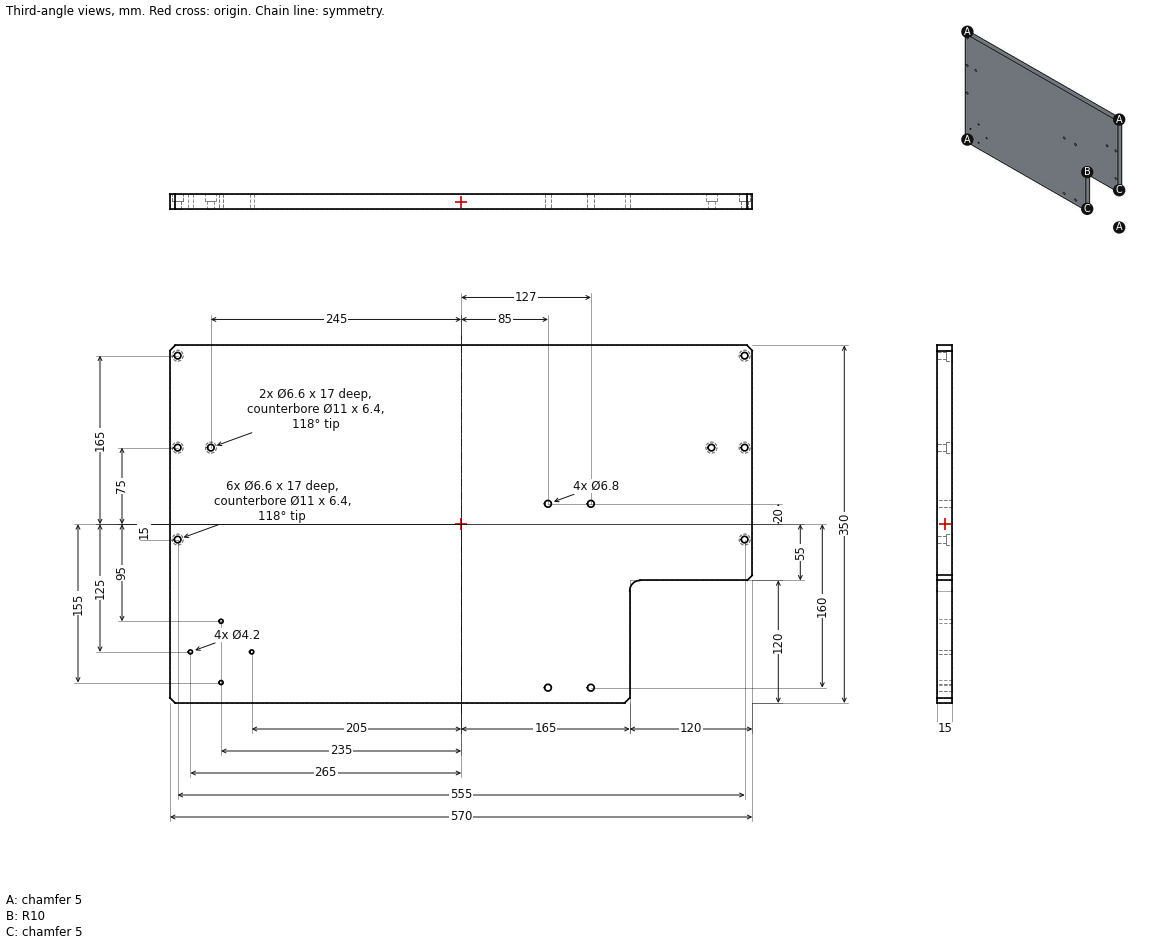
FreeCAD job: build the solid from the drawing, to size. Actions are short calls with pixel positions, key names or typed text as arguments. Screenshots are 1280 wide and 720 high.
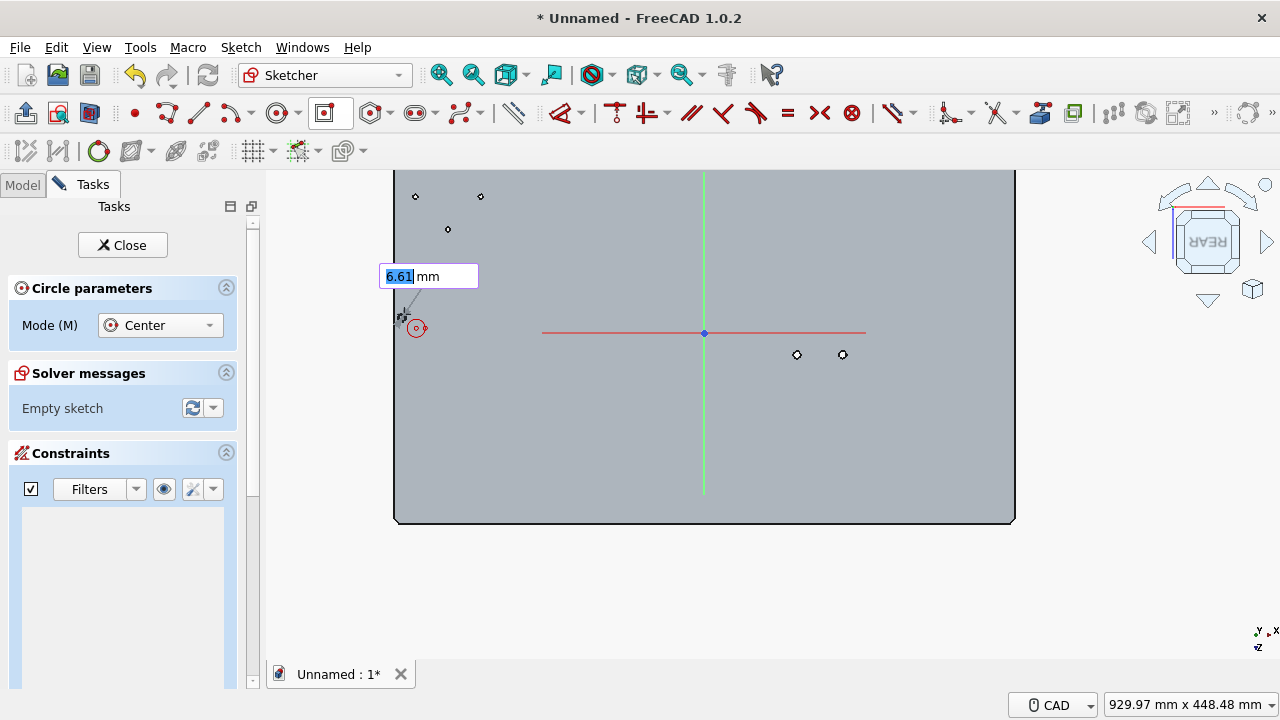
text(6.6)
key(Return)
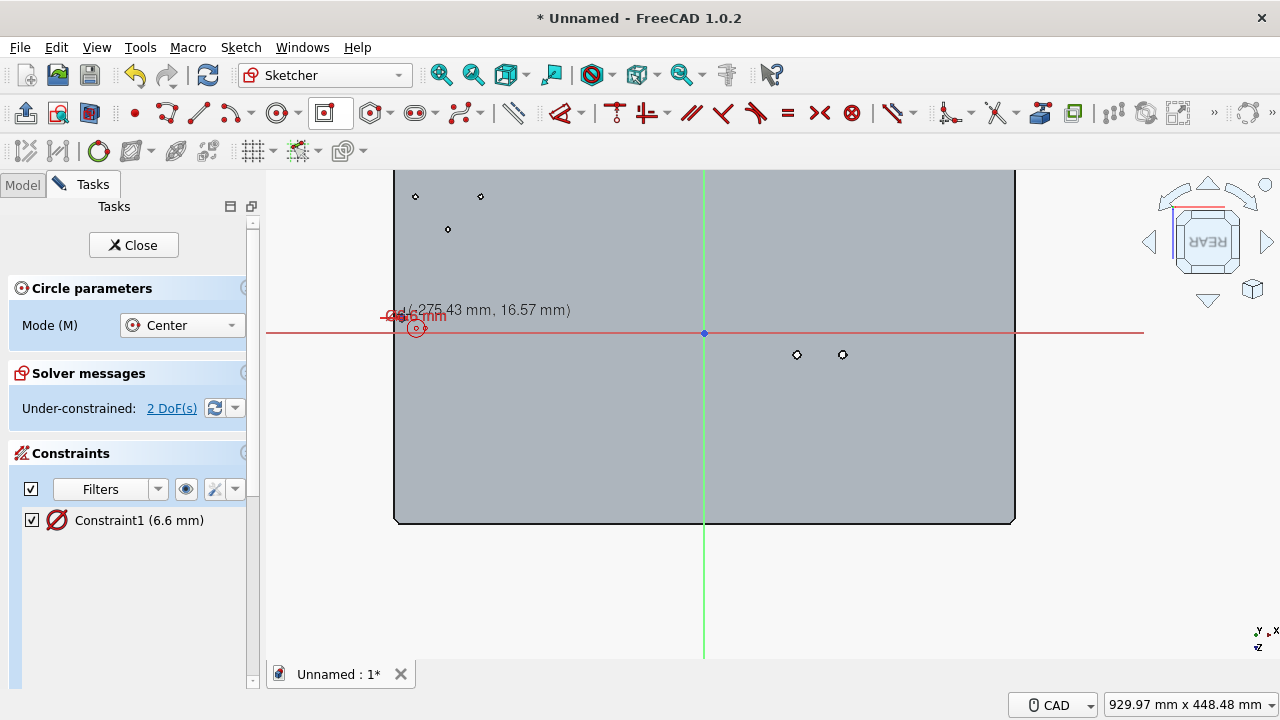
scroll(402, 513, up, 10)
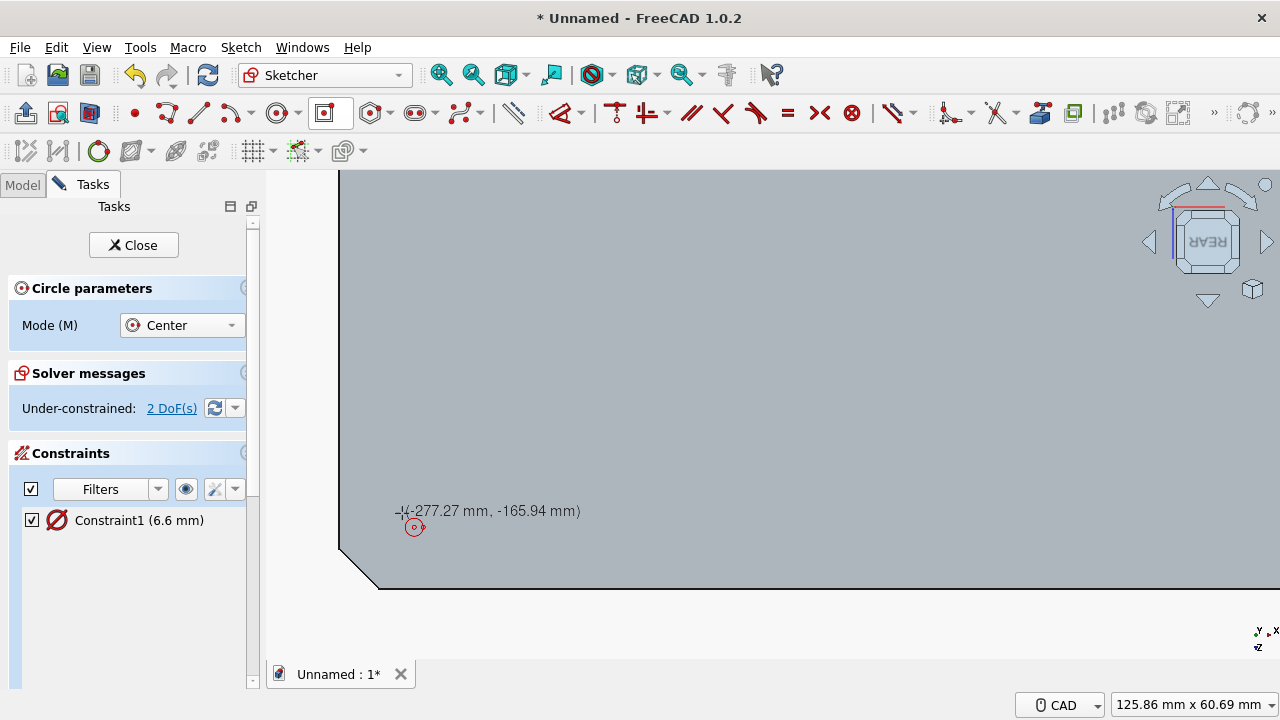
scroll(402, 513, down, 10)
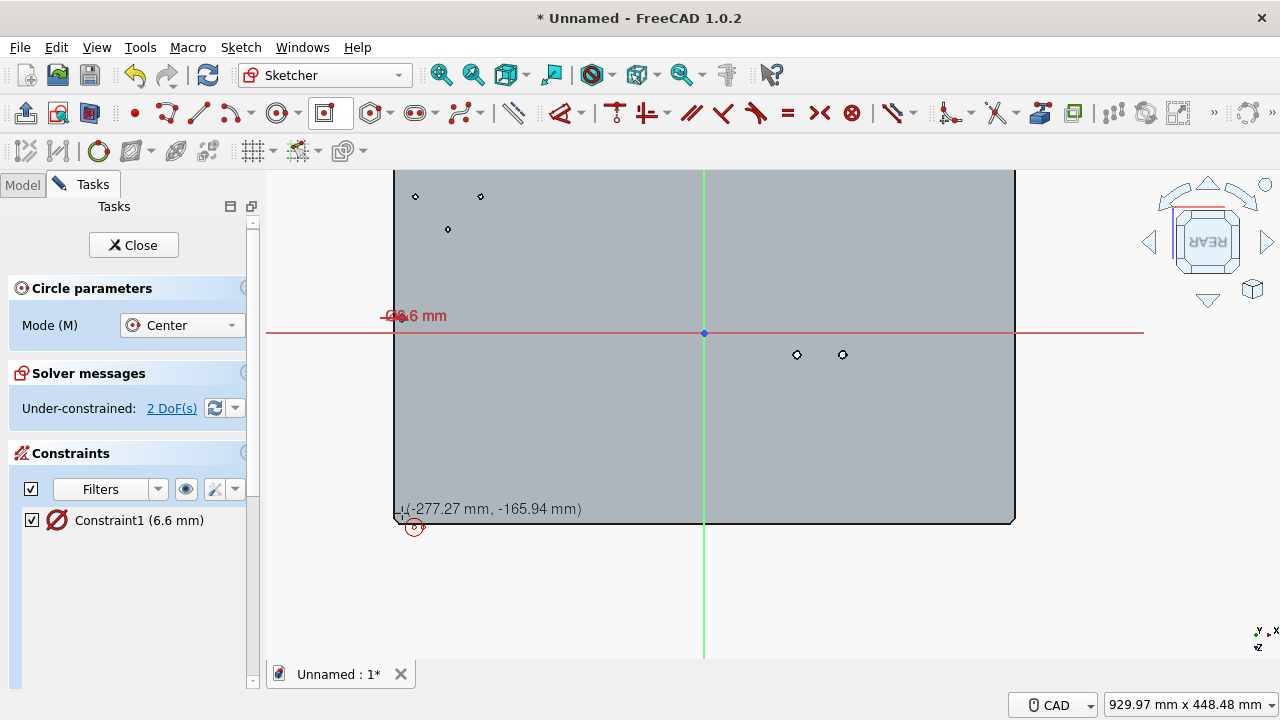
click(402, 513)
move(404, 510)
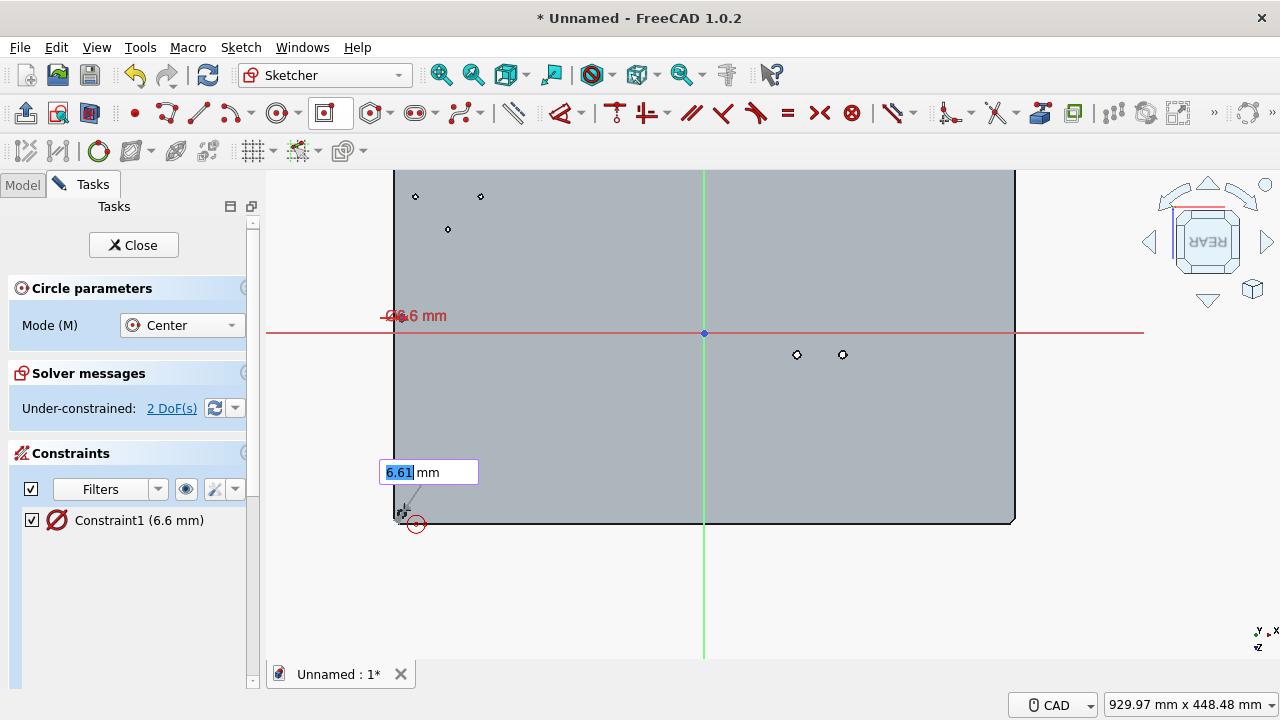
text(6.6)
key(Return)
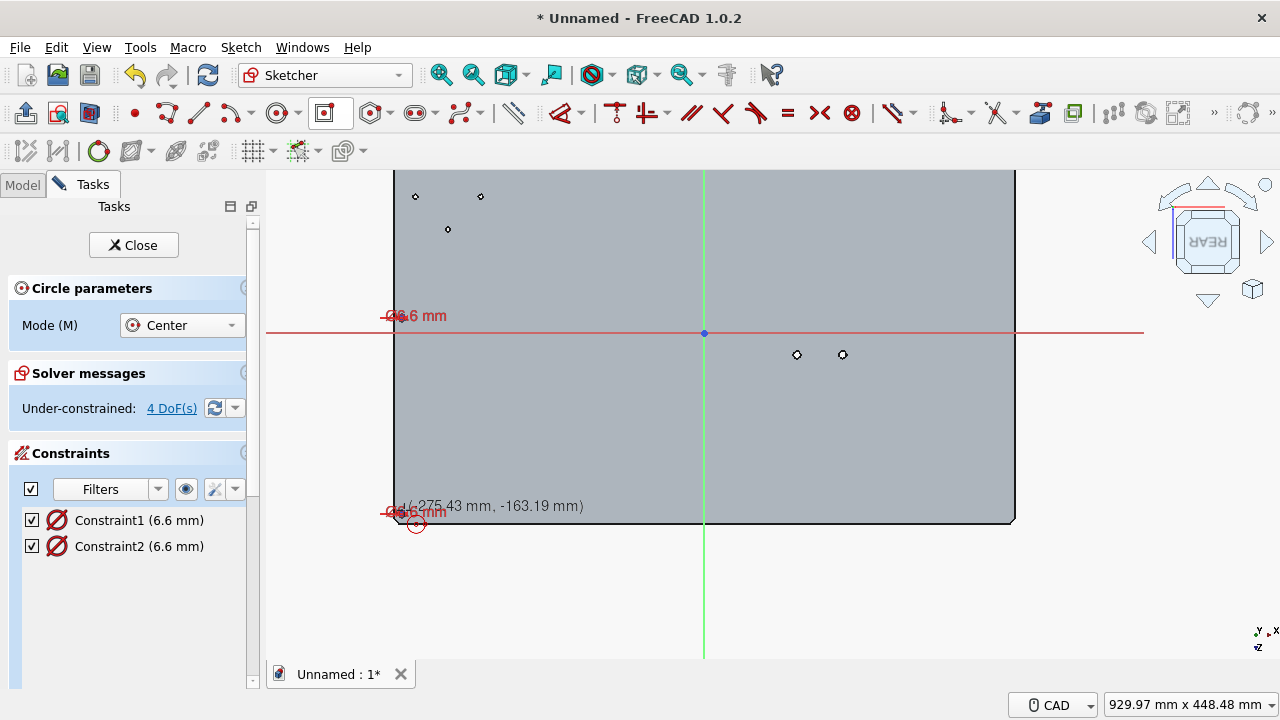
scroll(1007, 317, up, 10)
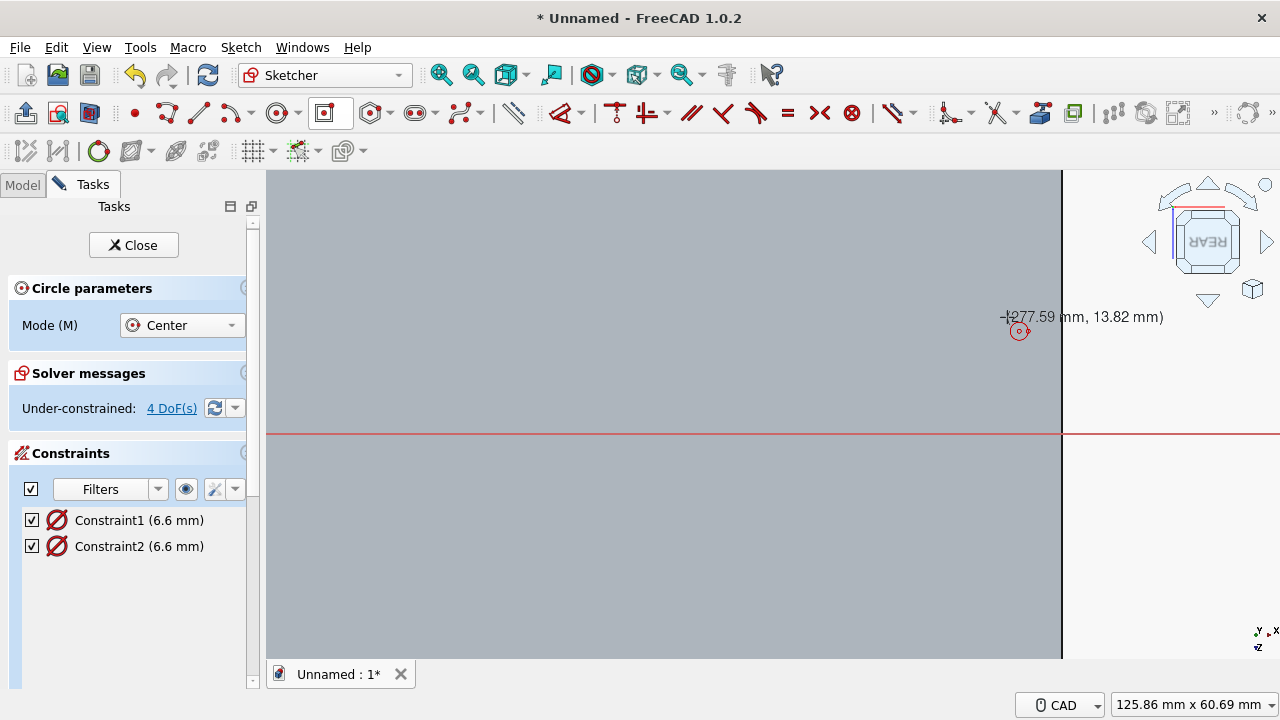
scroll(1008, 317, down, 10)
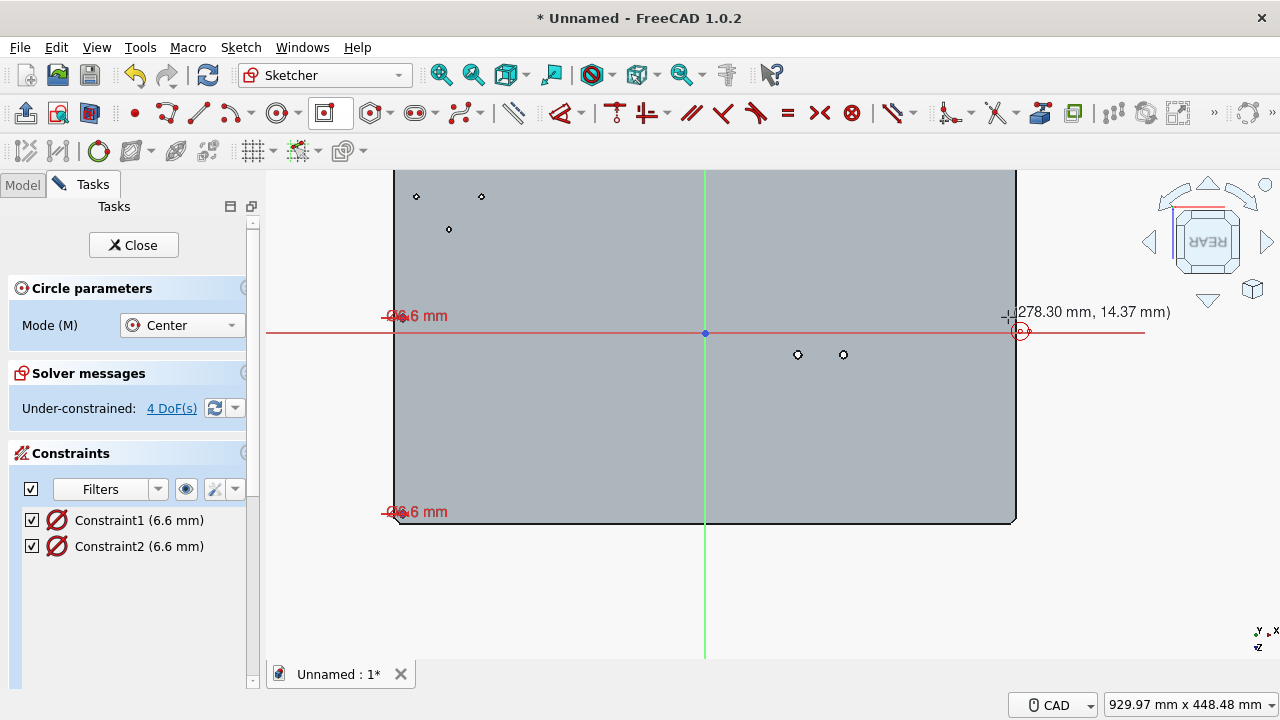
click(1008, 317)
move(1010, 314)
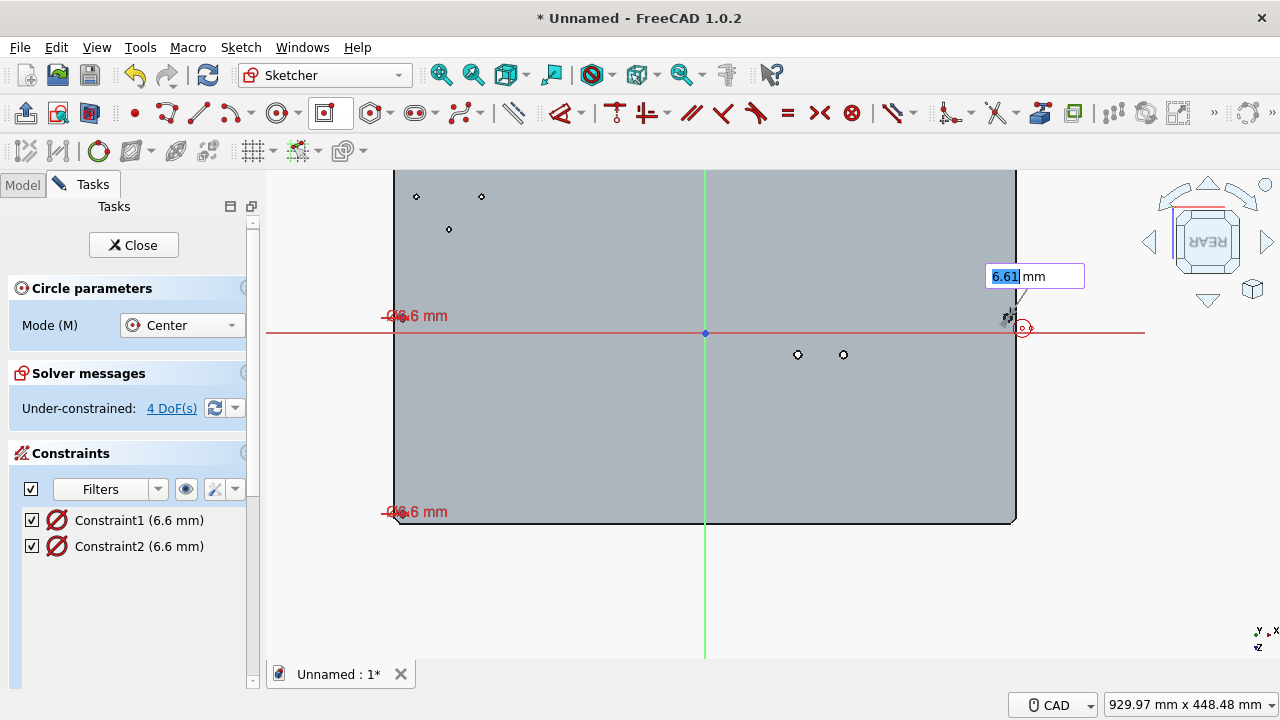
text(6.6)
key(Return)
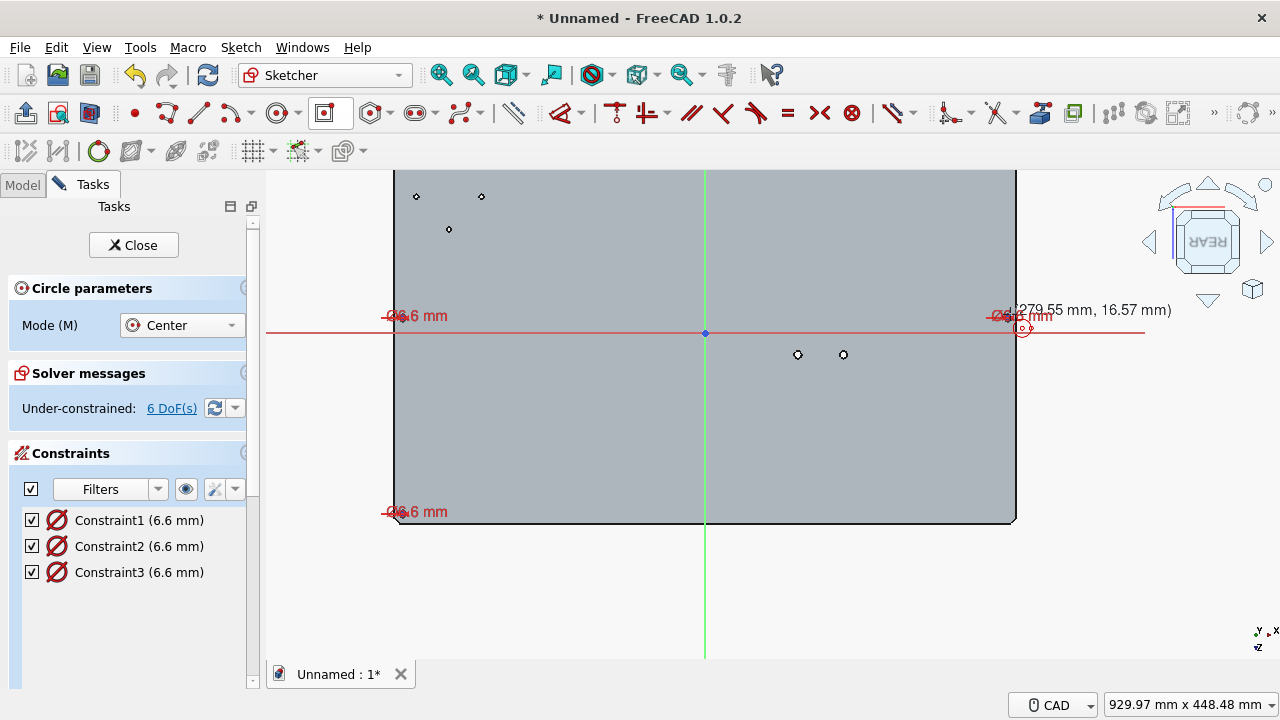
scroll(1008, 513, up, 10)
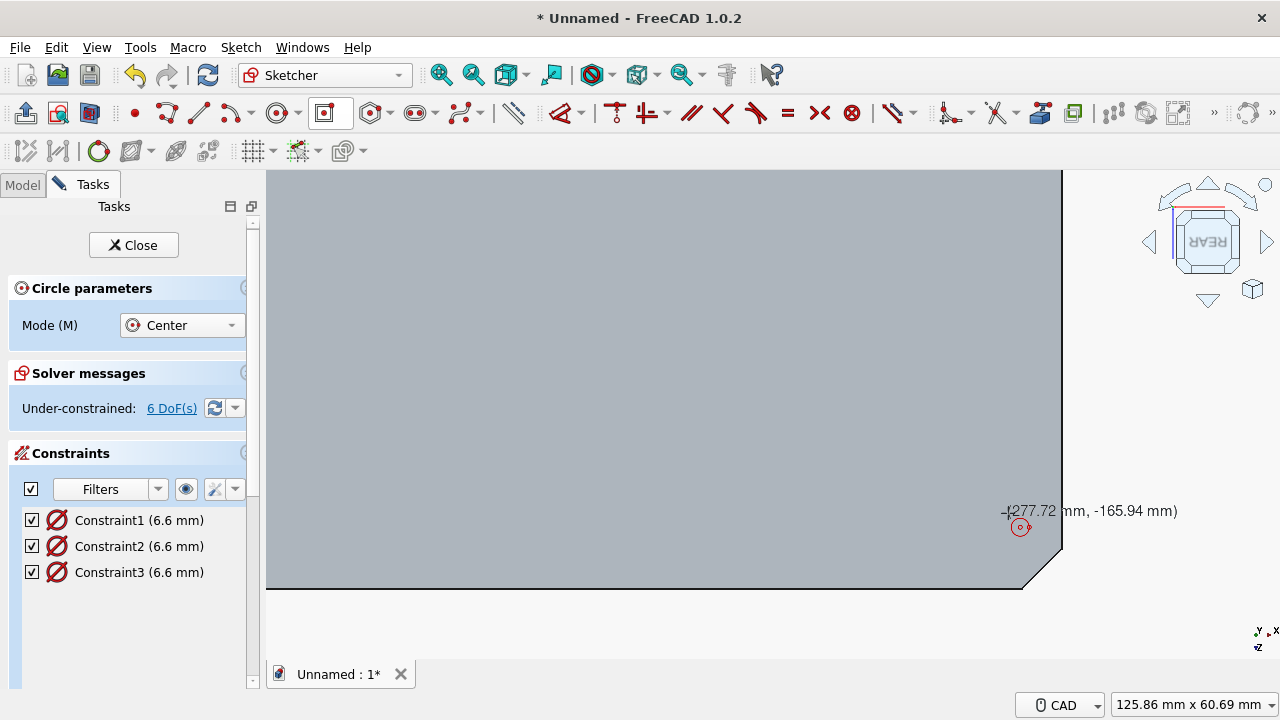
scroll(1008, 513, down, 10)